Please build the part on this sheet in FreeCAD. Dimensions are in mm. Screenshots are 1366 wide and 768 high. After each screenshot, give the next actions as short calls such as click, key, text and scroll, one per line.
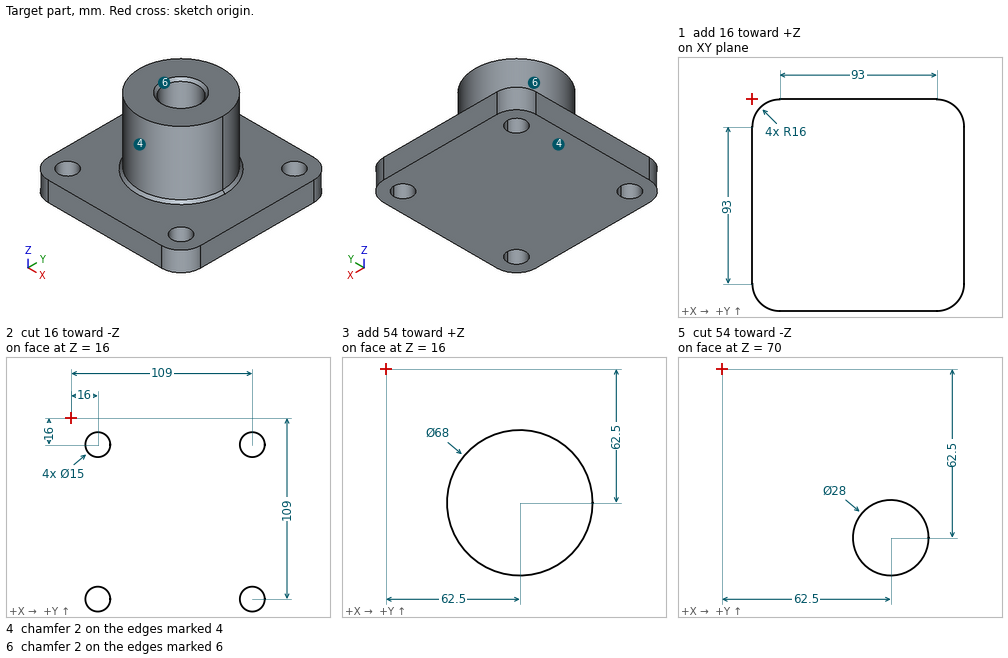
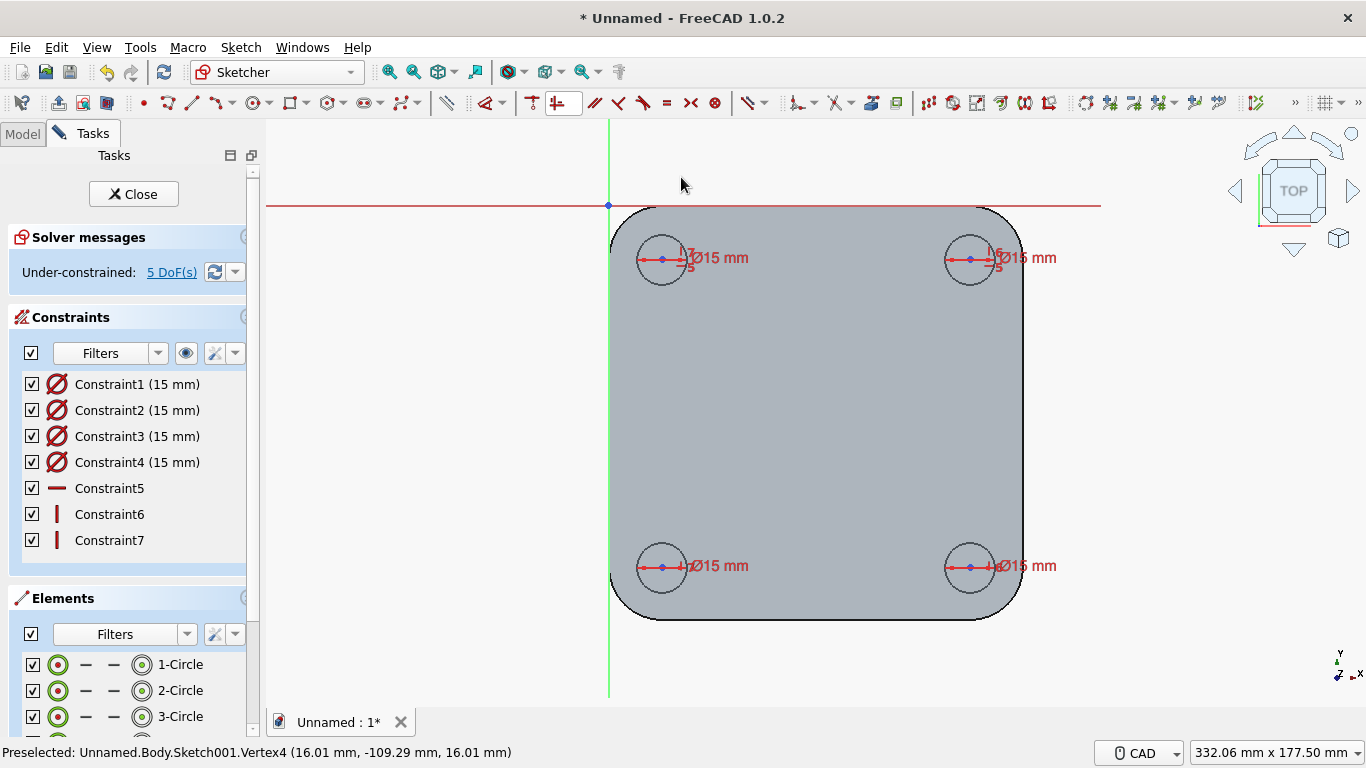
click(970, 568)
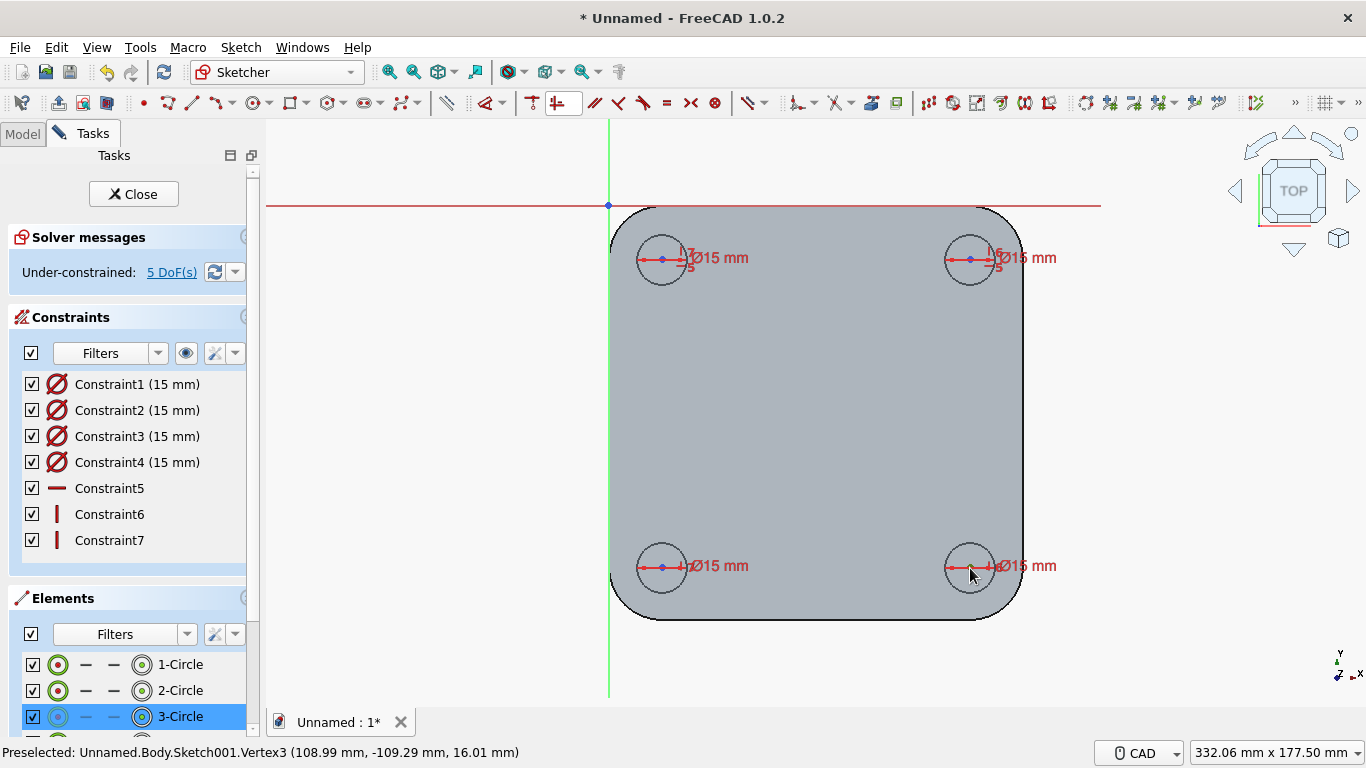
click(662, 568)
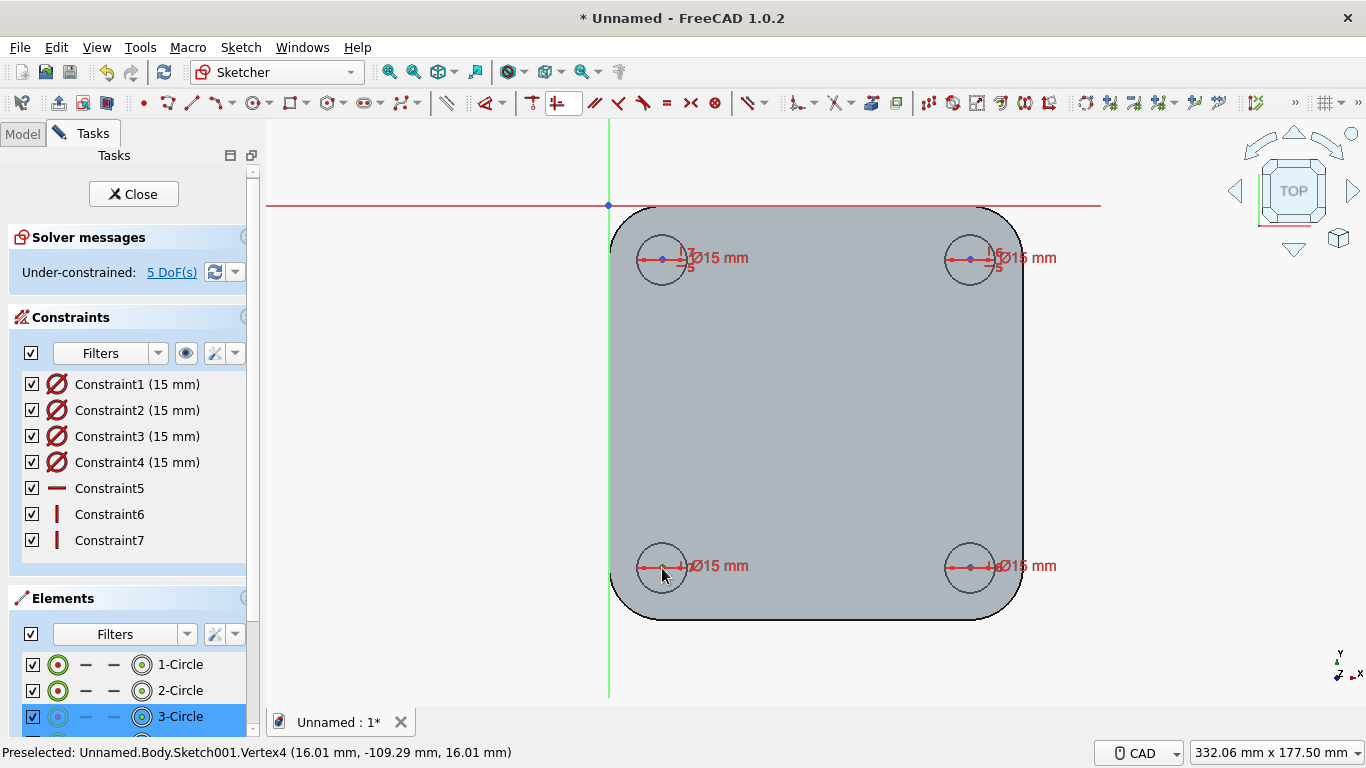
key(h)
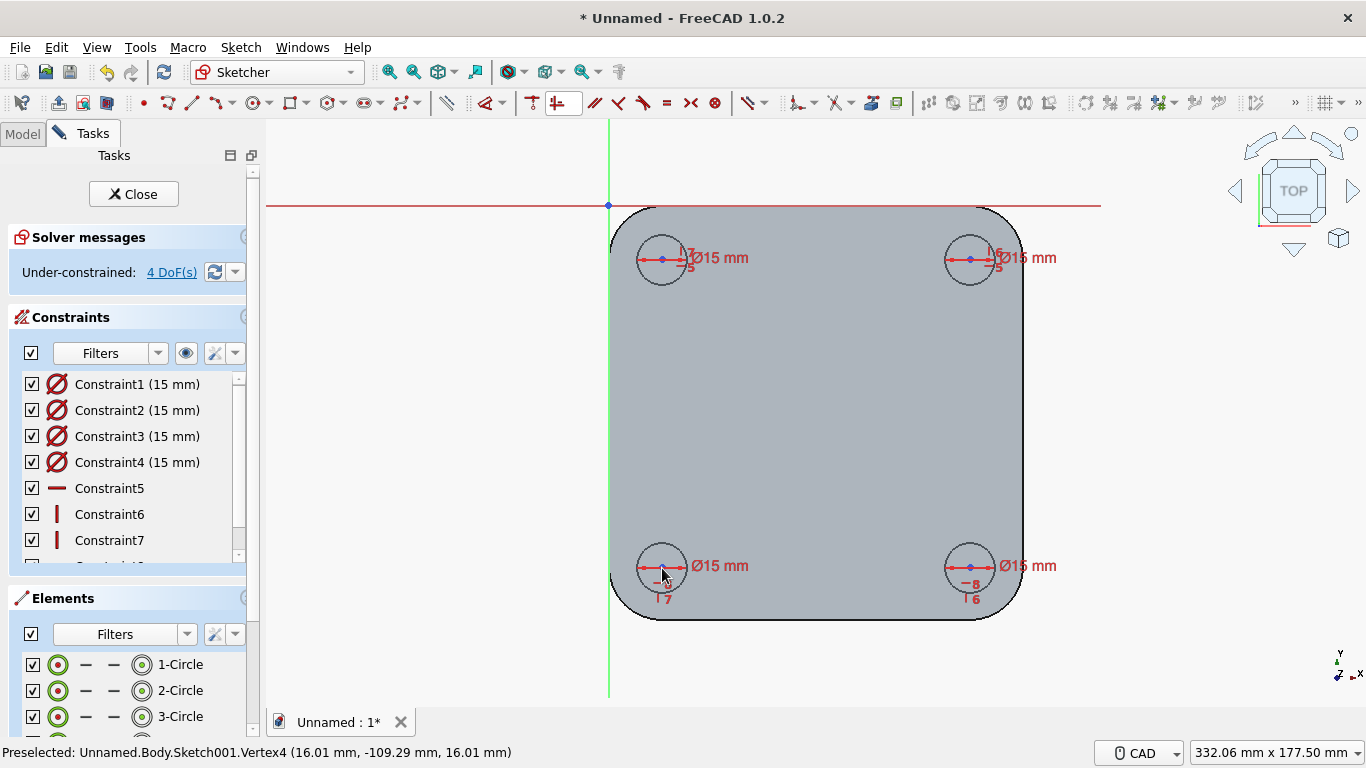
click(486, 104)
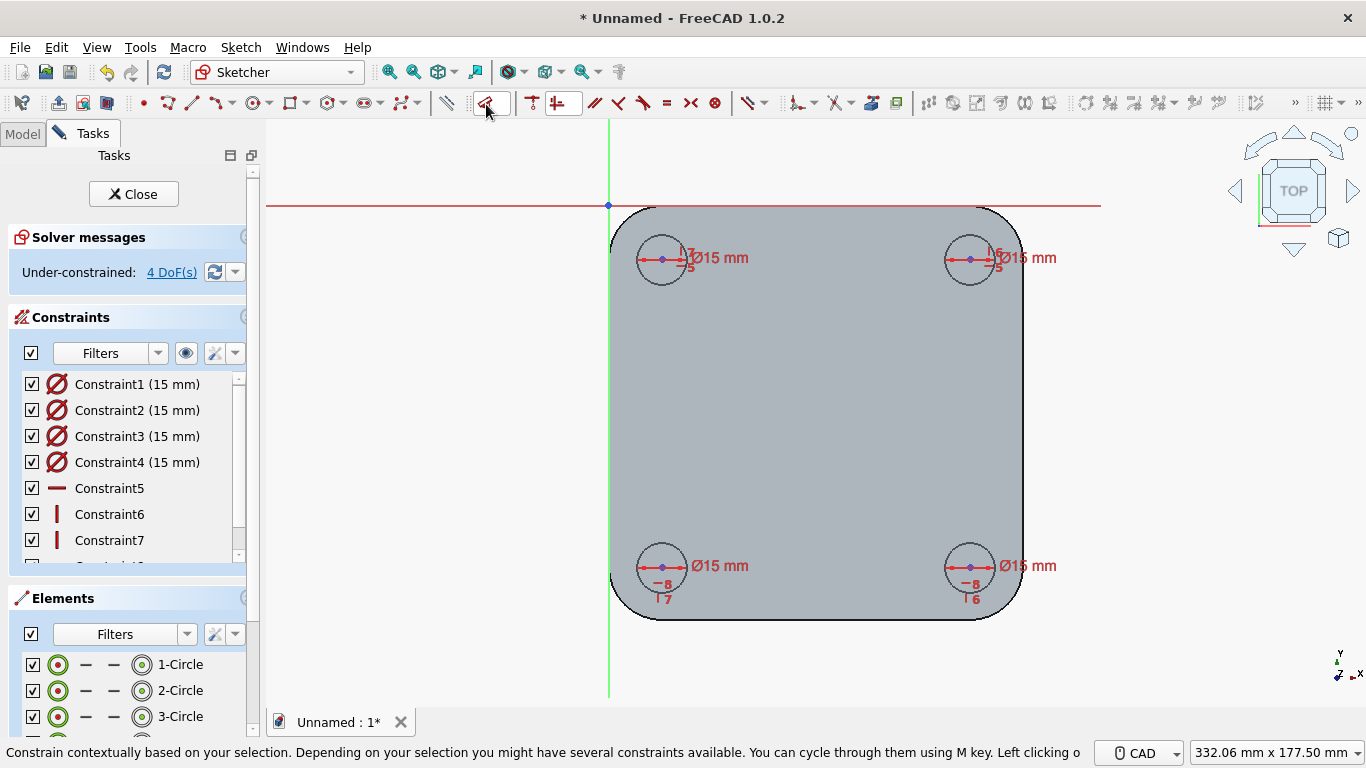
click(662, 260)
click(635, 172)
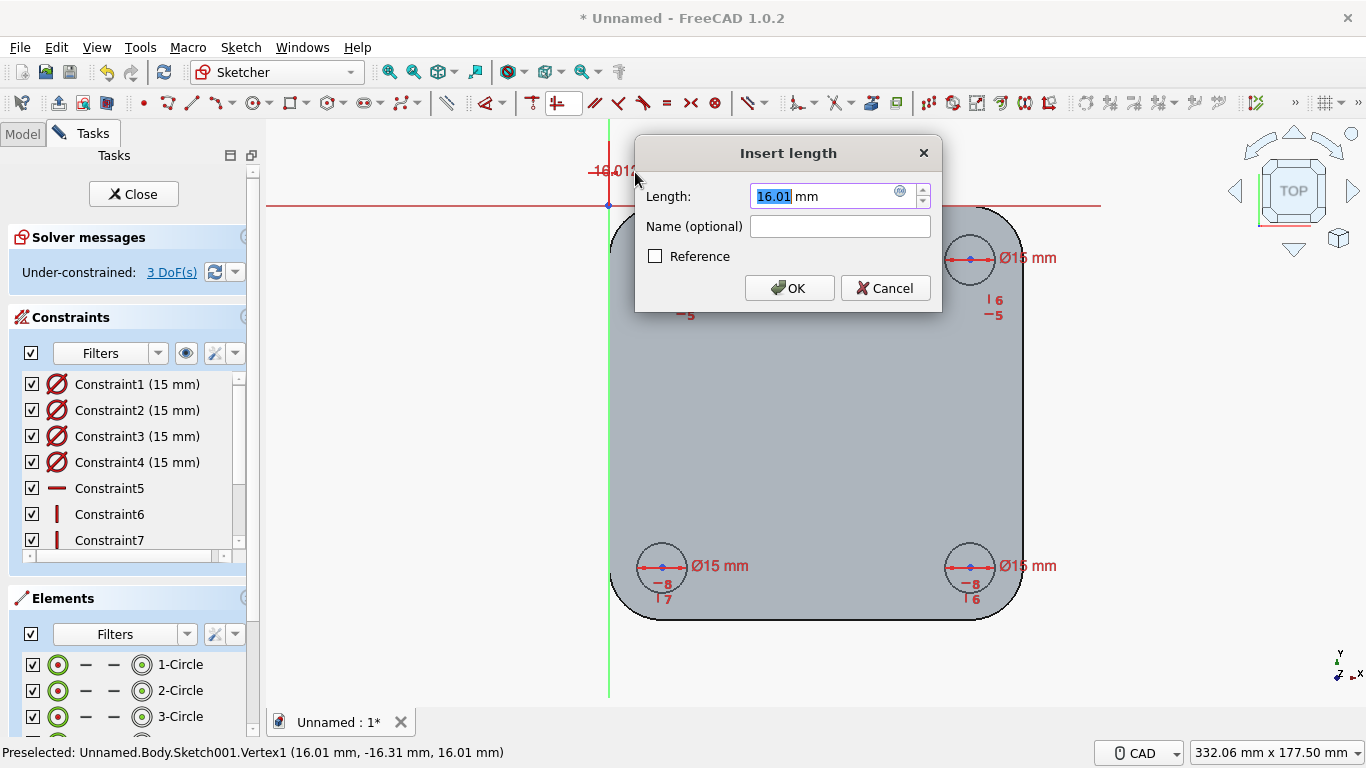
text(16)
key(Return)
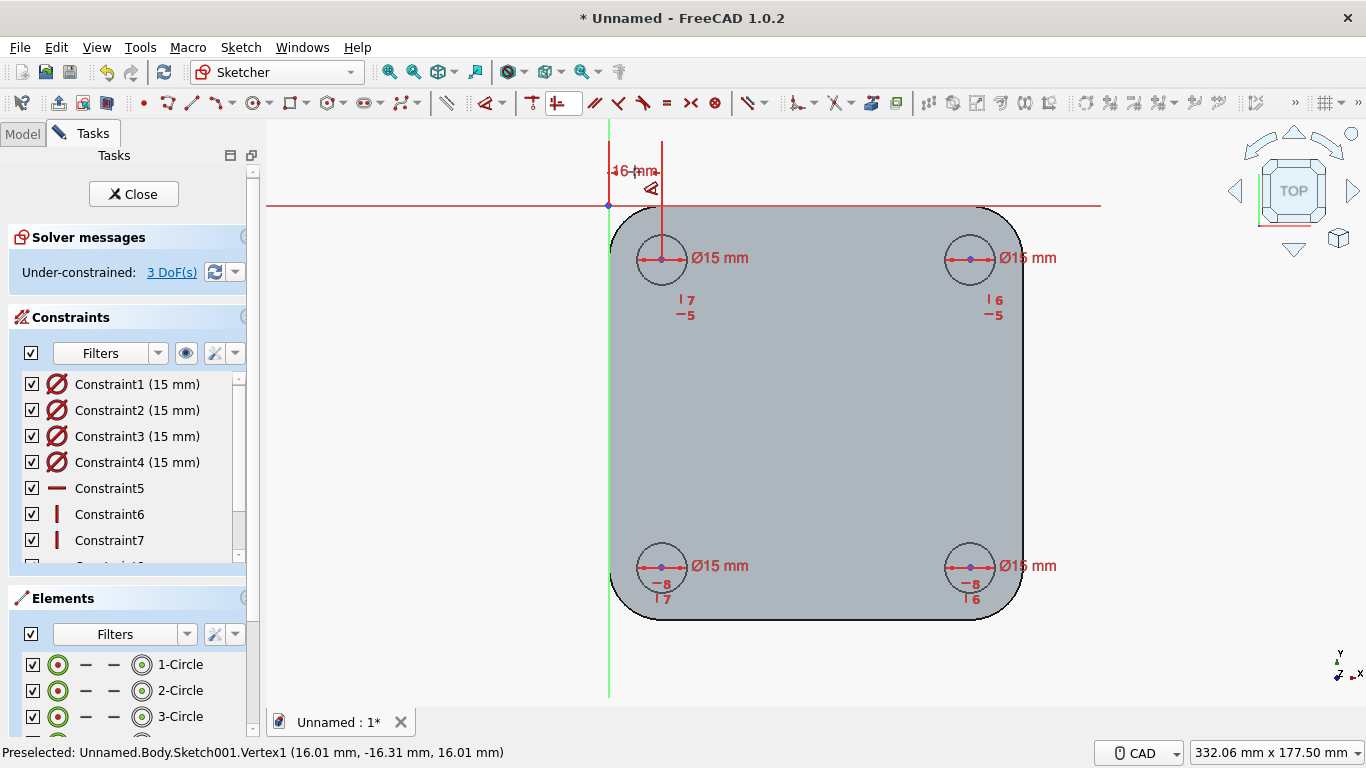
click(662, 260)
click(575, 233)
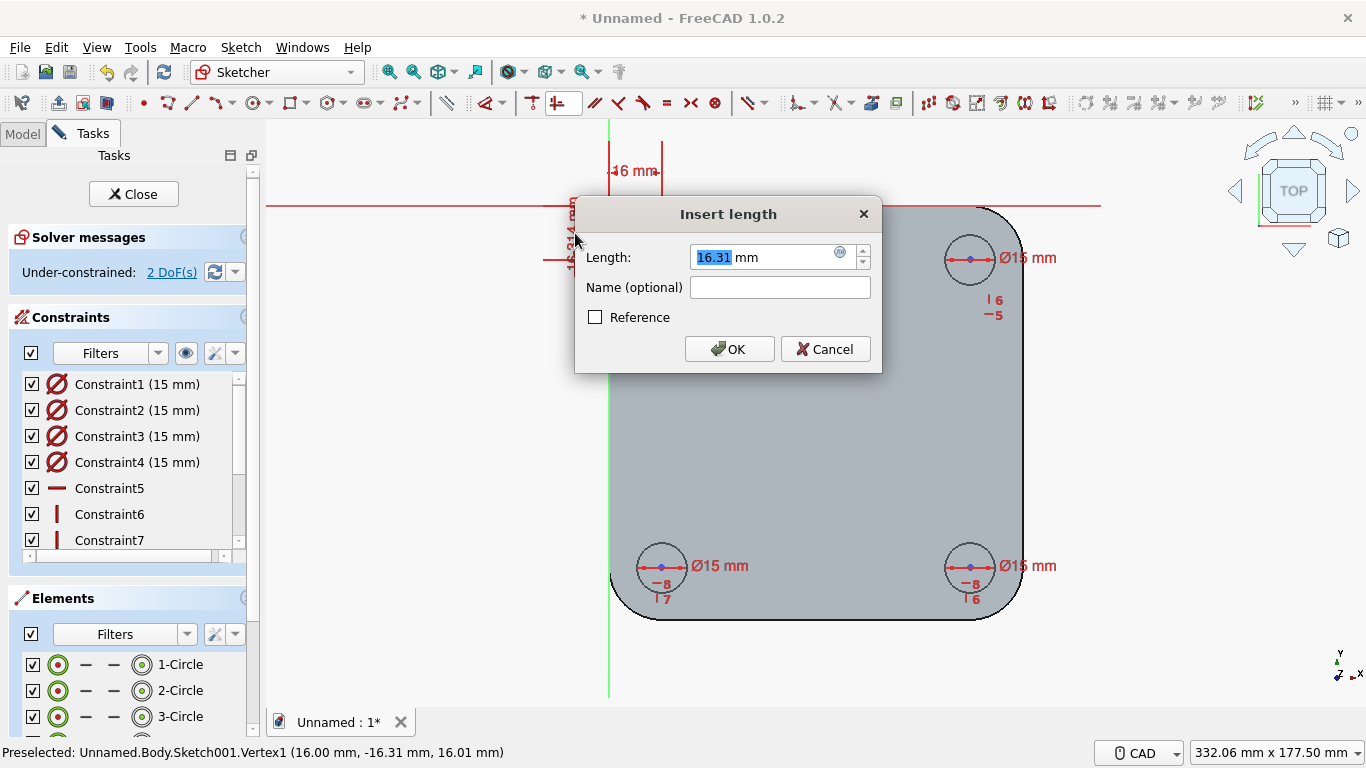
text(16)
key(Return)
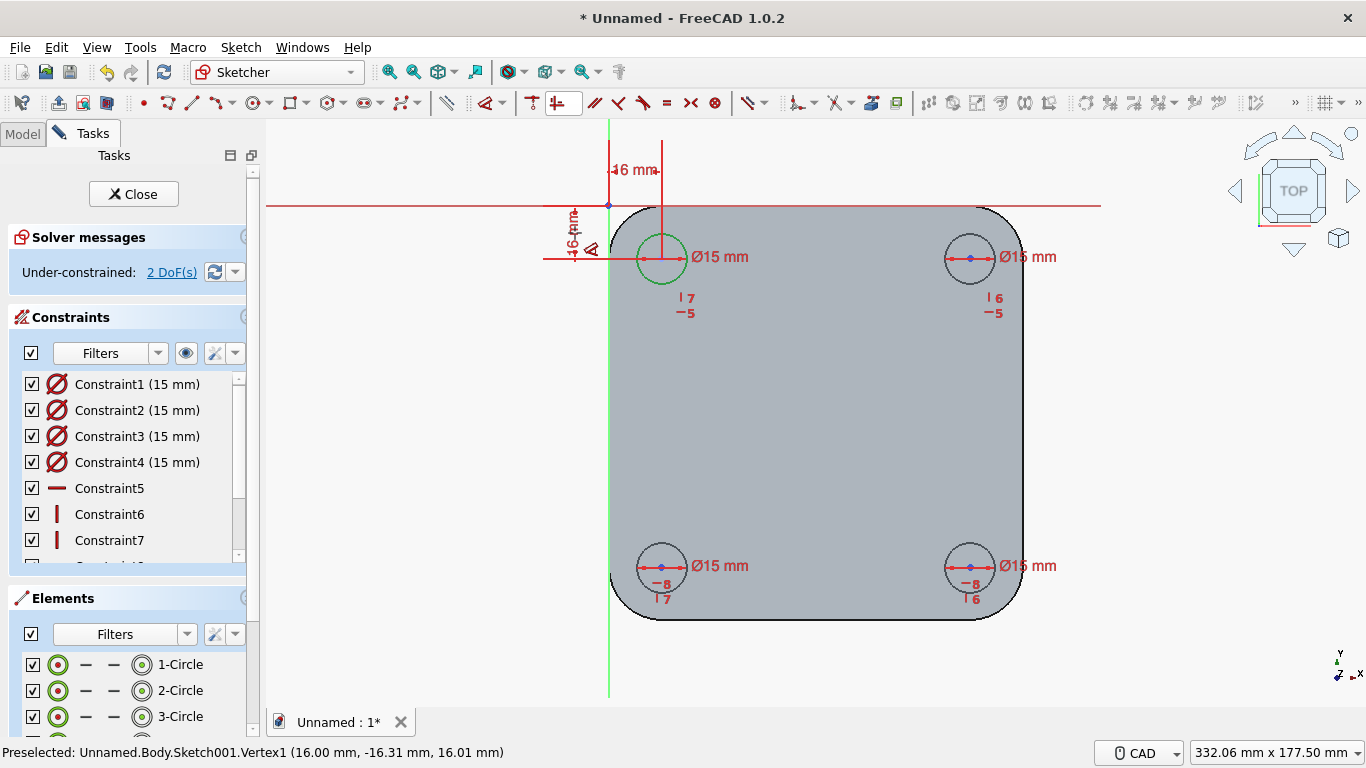
click(970, 259)
click(789, 172)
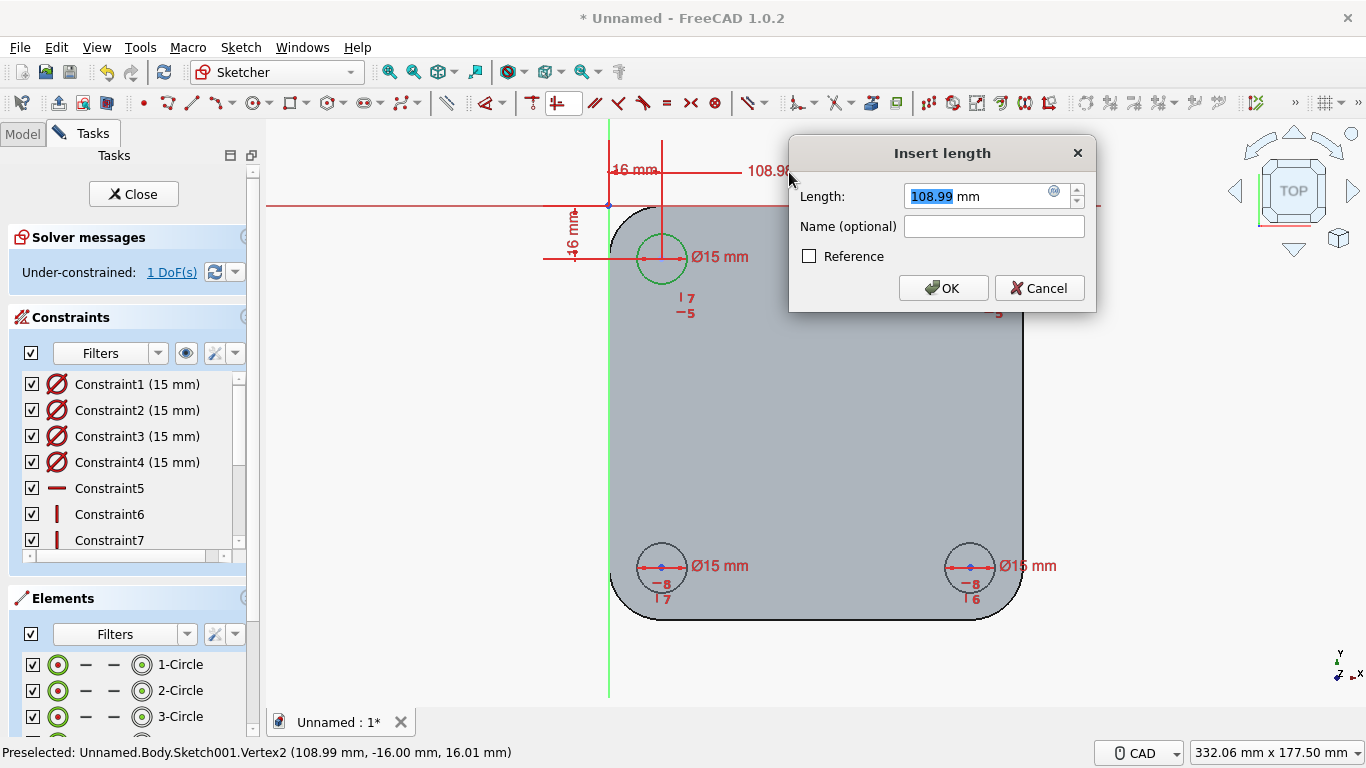
text(109)
key(Return)